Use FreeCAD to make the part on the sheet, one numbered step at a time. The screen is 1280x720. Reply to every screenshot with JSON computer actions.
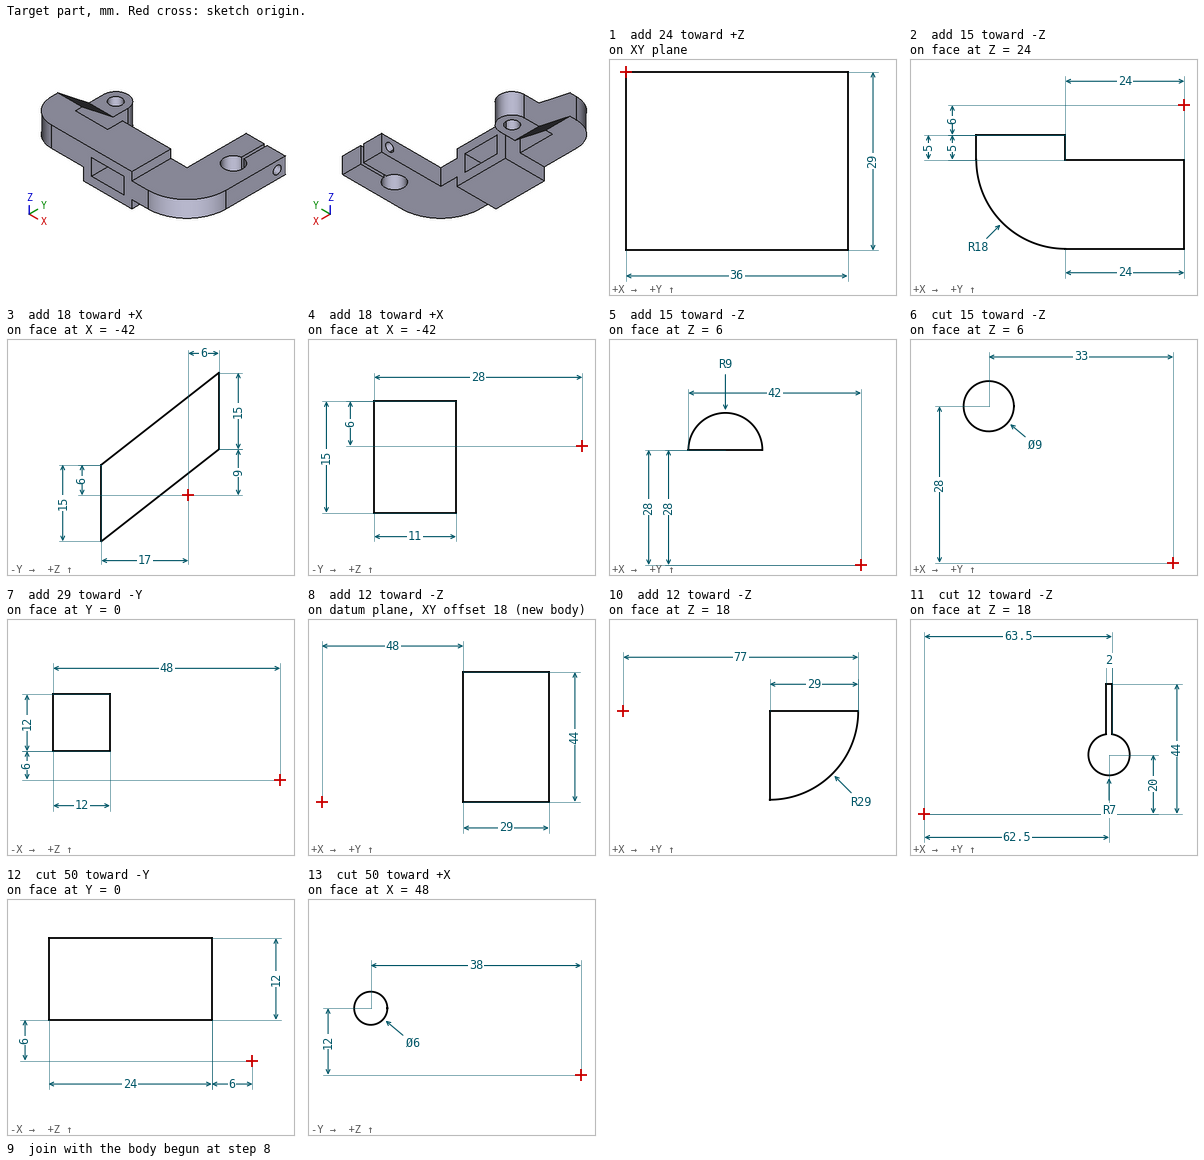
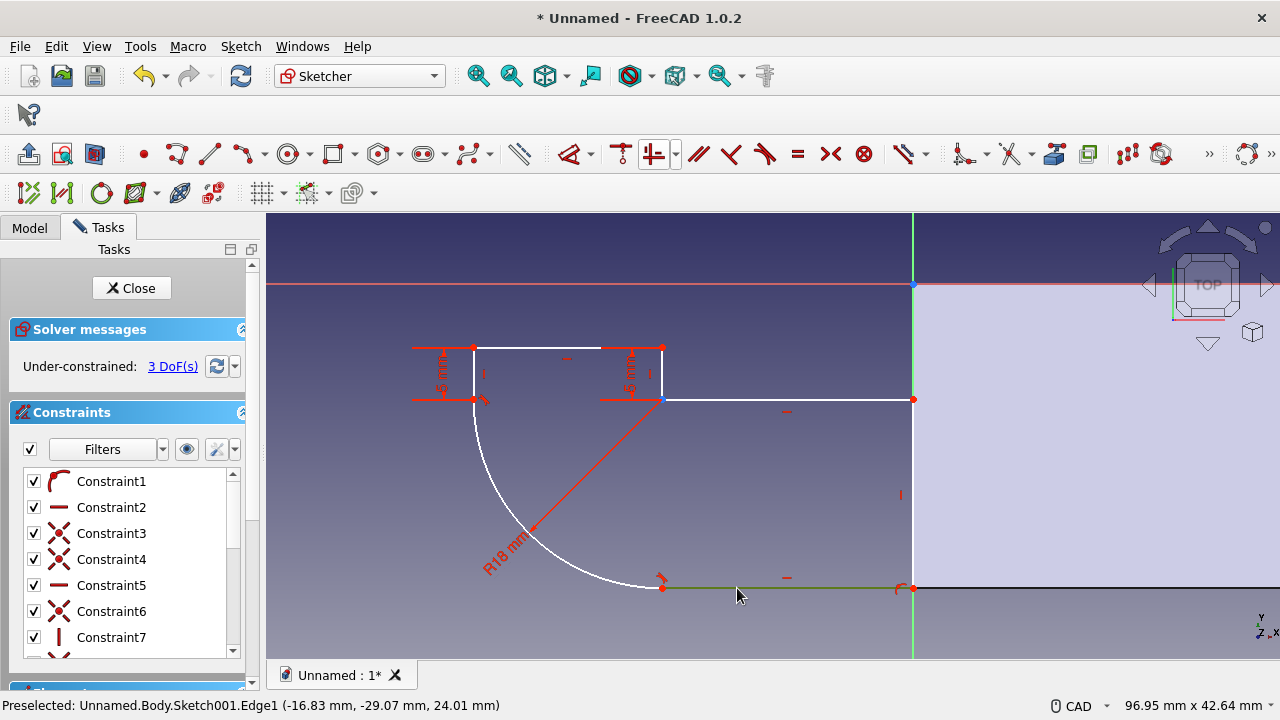
{"action": "key", "text": "l"}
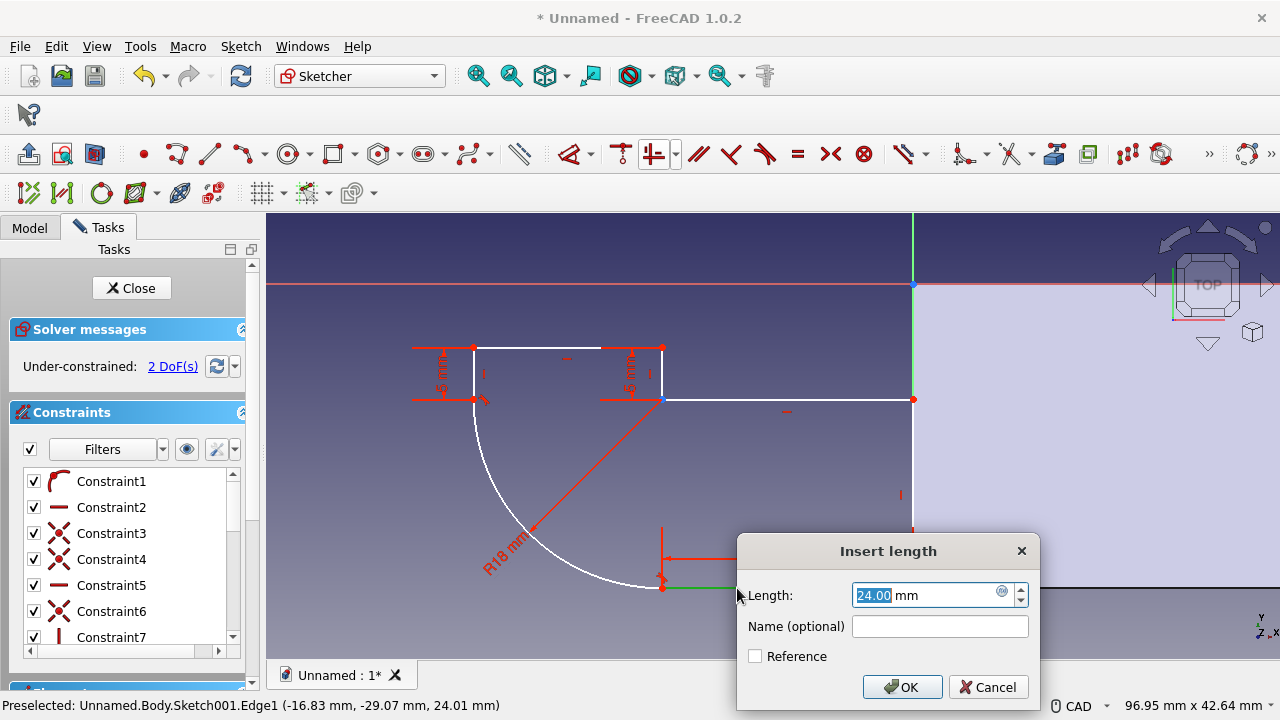
{"action": "type", "text": "24"}
{"action": "key", "text": "Return"}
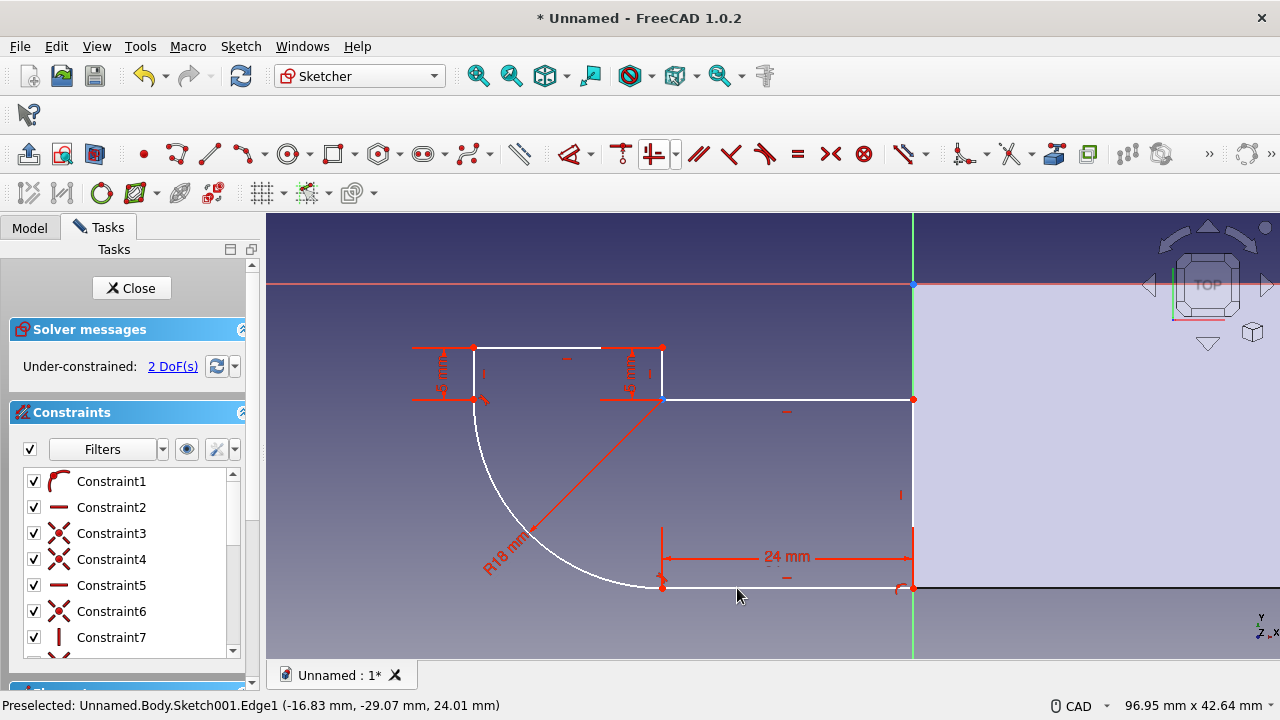
{"action": "left_click", "coordinate": [838, 400]}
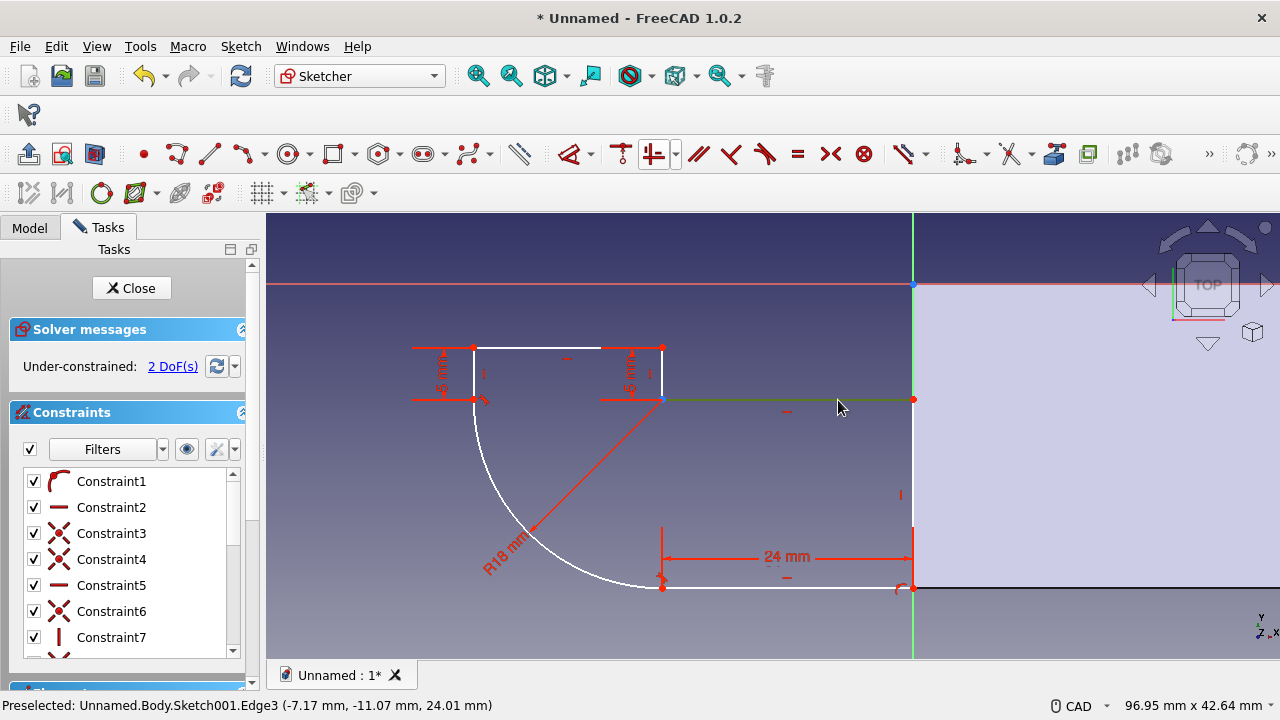
{"action": "key", "text": "l"}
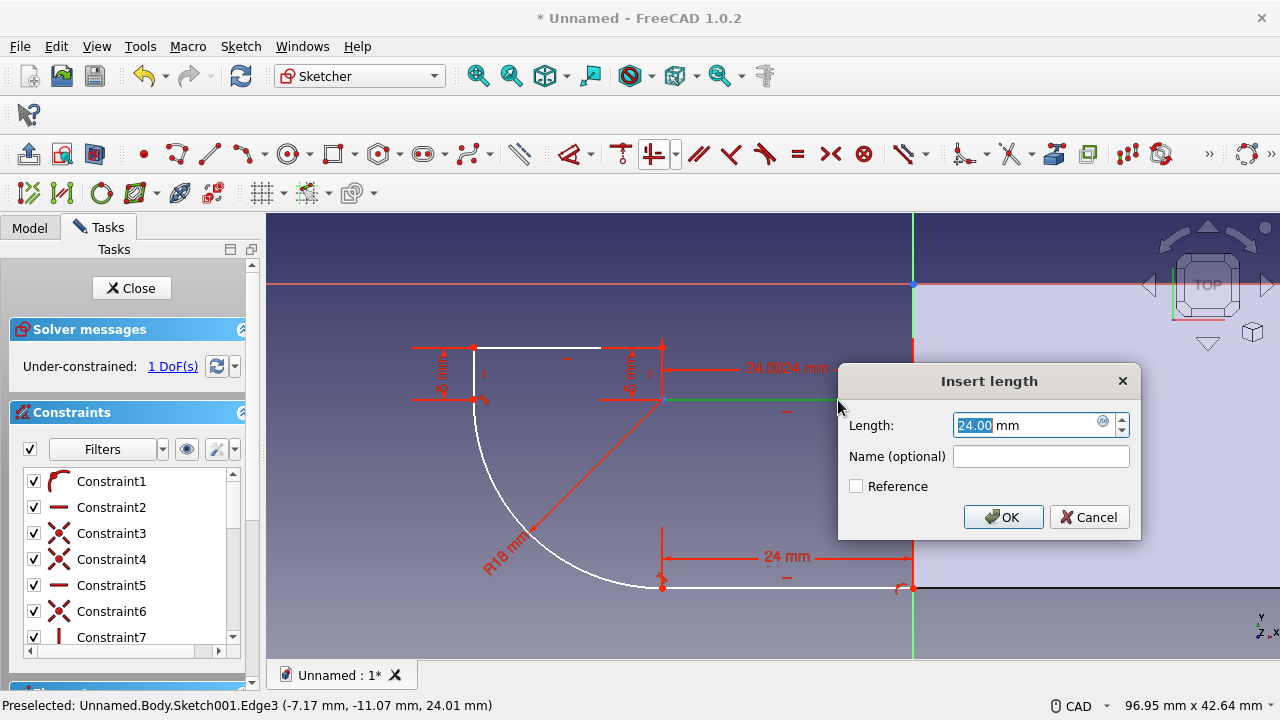
{"action": "type", "text": "24"}
{"action": "key", "text": "Return"}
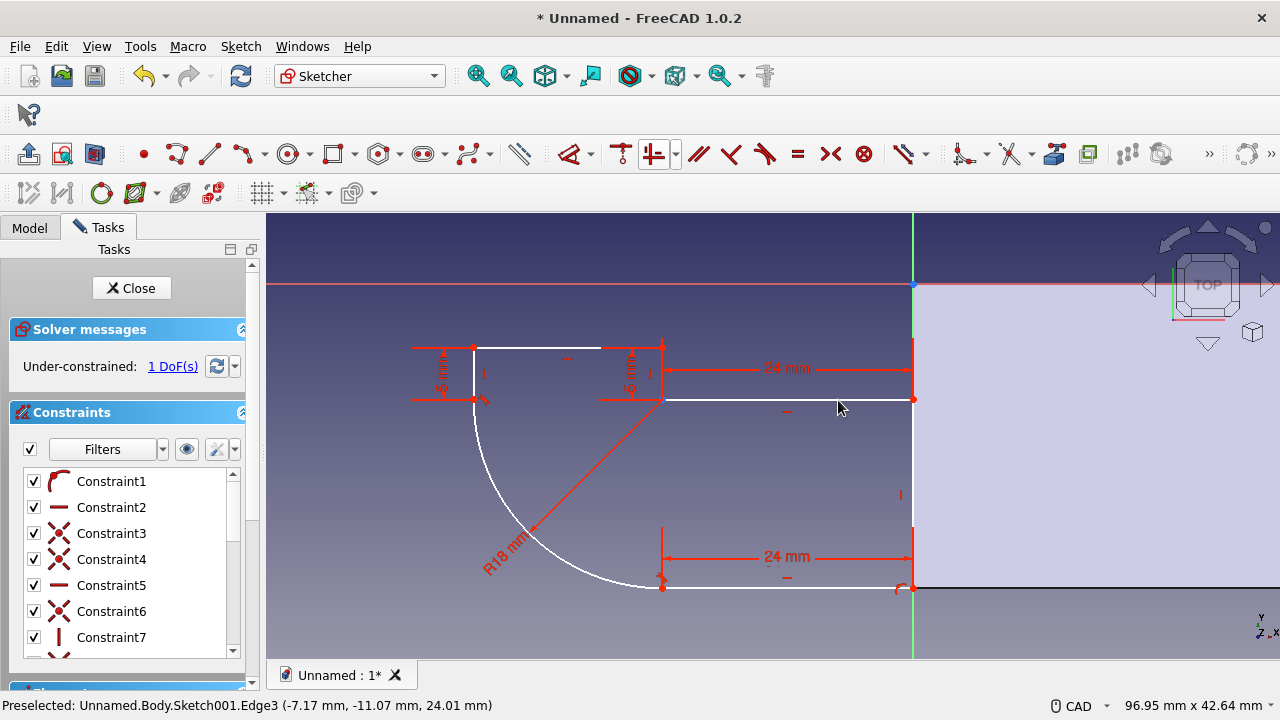
{"action": "left_click", "coordinate": [662, 348]}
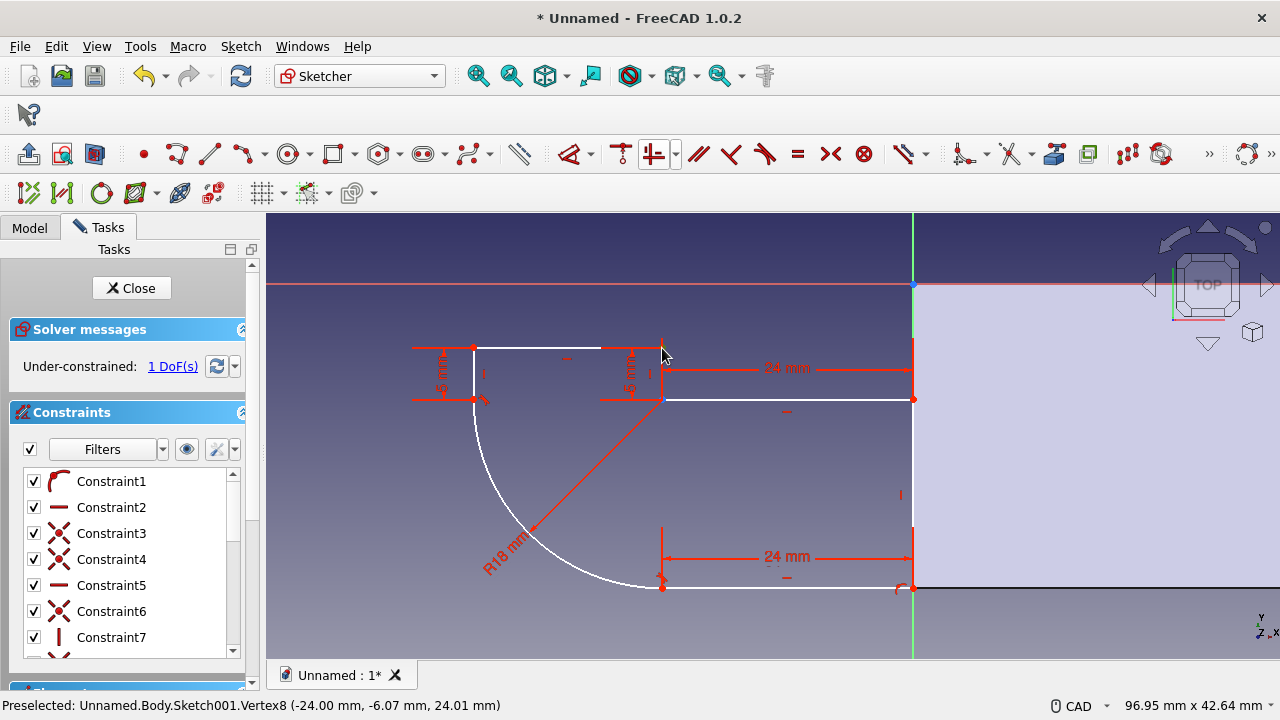
{"action": "left_click", "coordinate": [590, 154]}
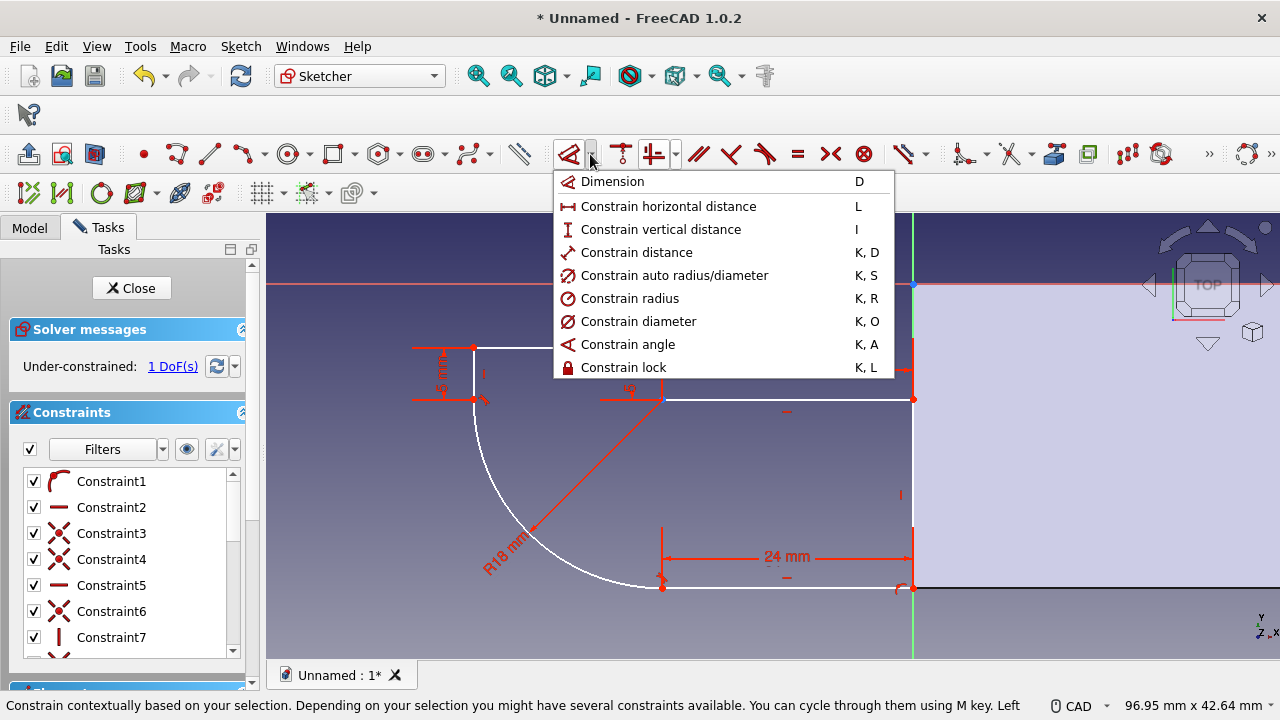
{"action": "left_click", "coordinate": [724, 230]}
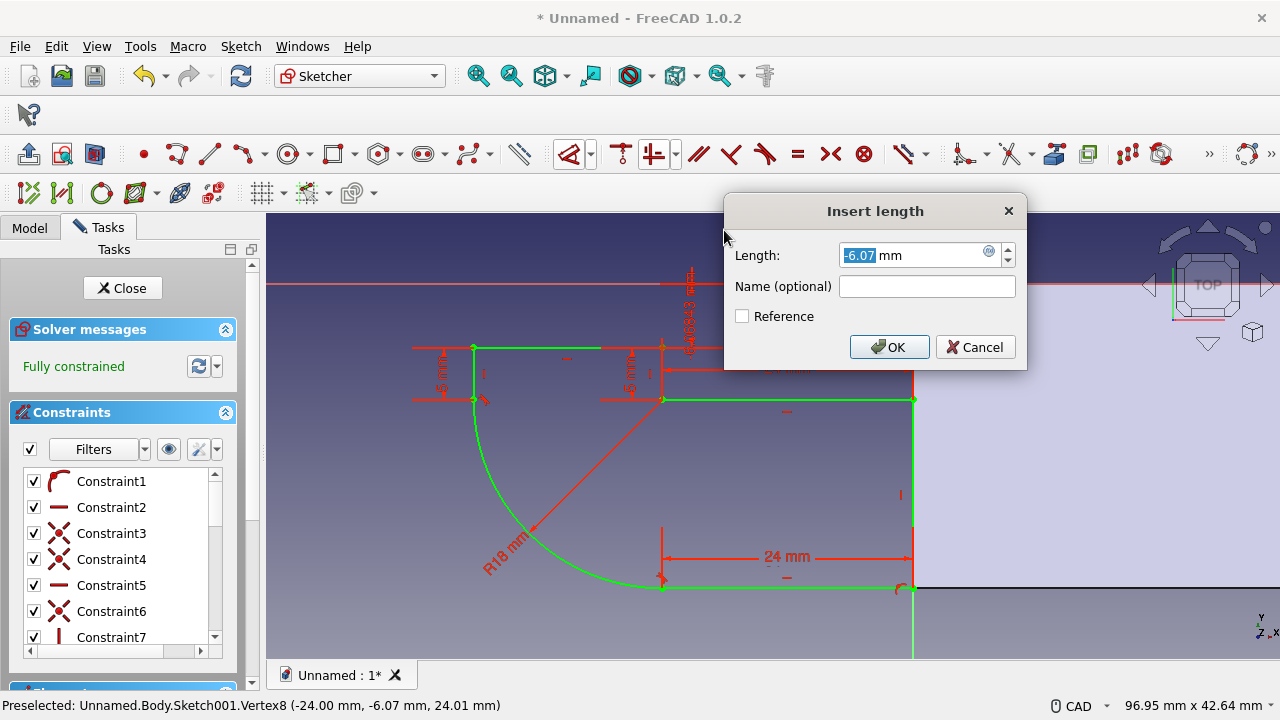
{"action": "type", "text": "-6"}
{"action": "key", "text": "Return"}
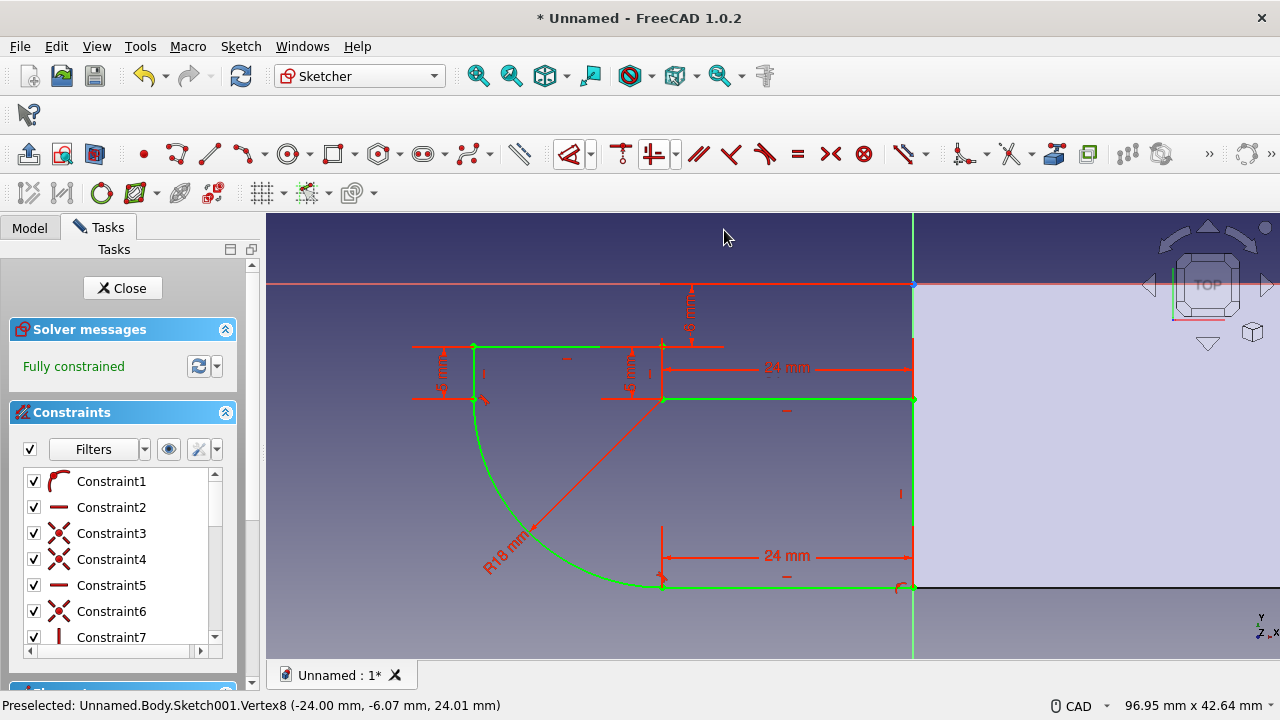
{"action": "left_click", "coordinate": [123, 288]}